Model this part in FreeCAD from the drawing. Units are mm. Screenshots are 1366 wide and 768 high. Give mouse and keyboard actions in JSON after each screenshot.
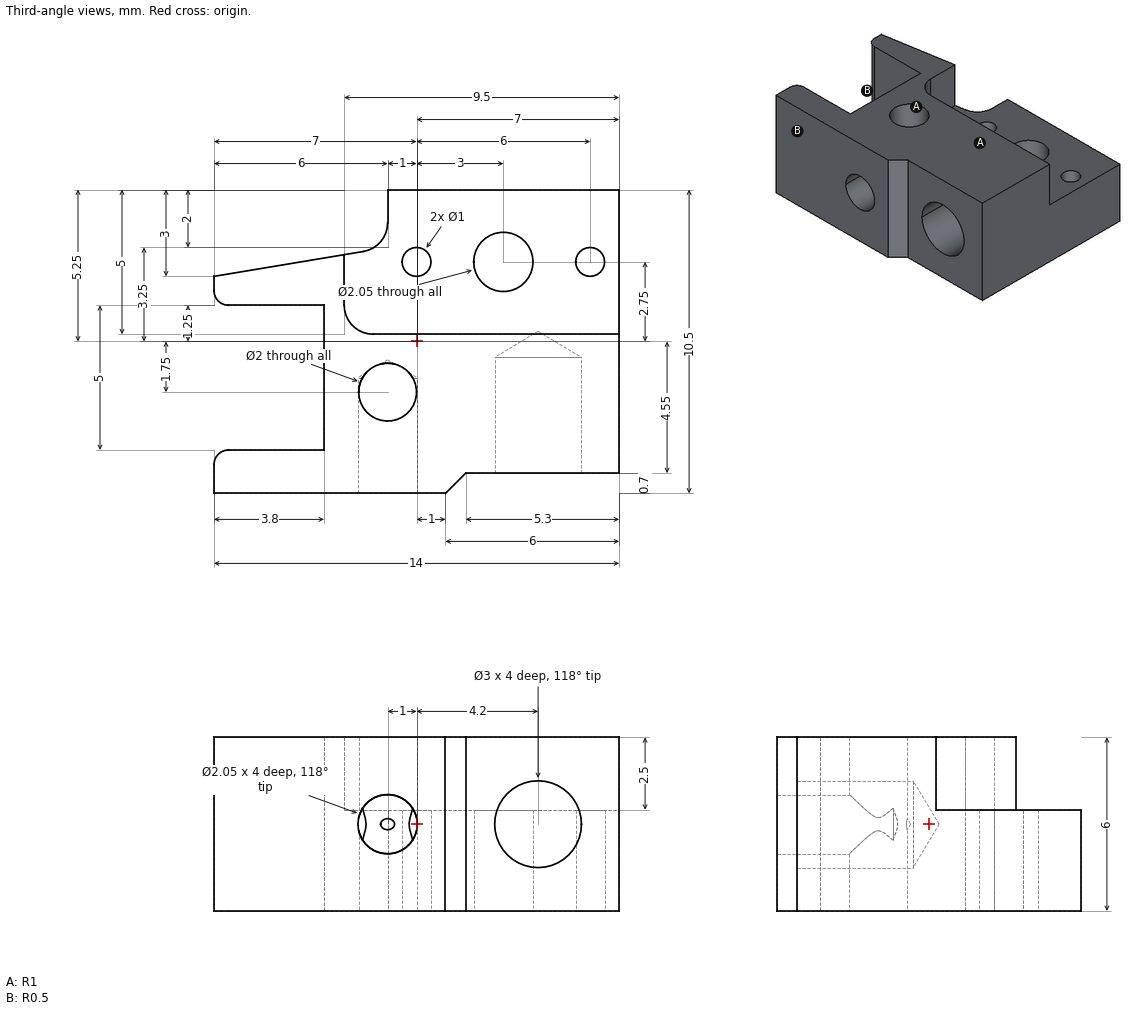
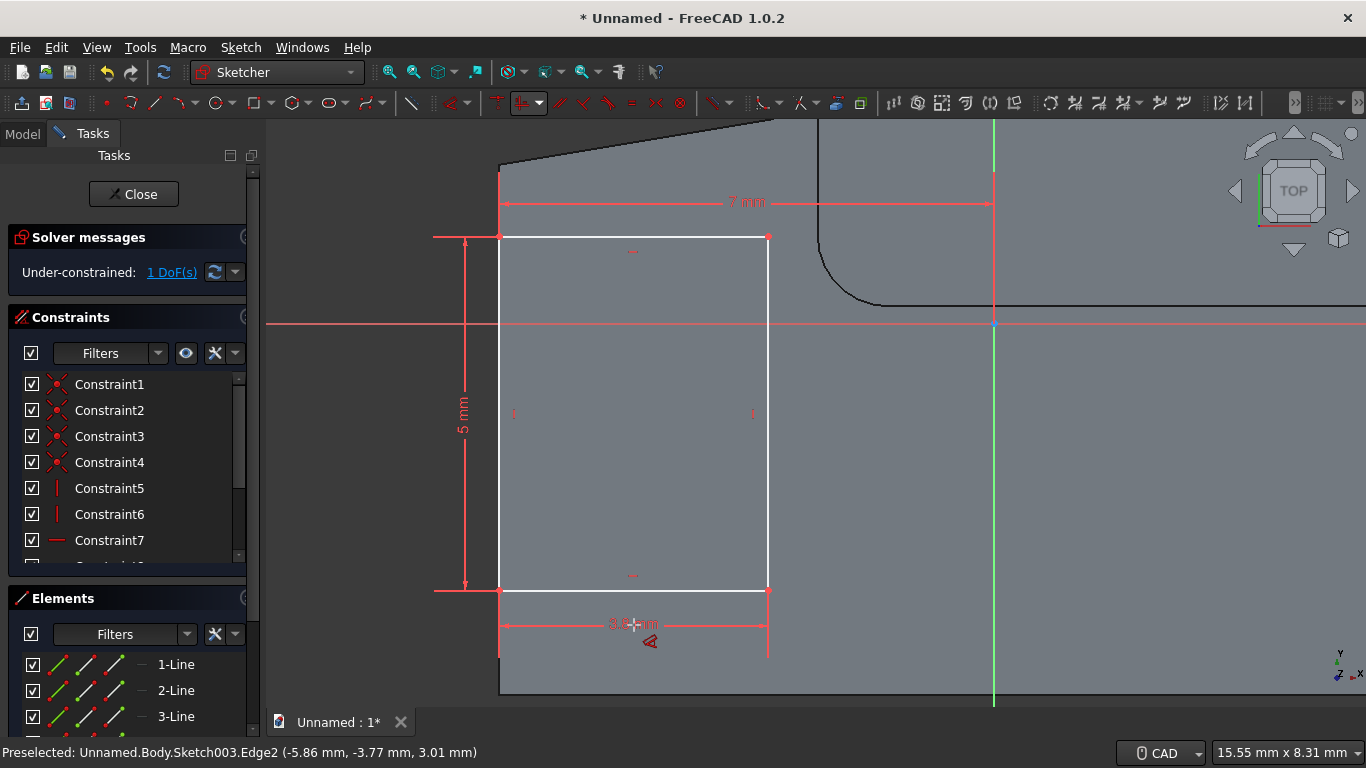
{"action": "left_click", "coordinate": [499, 237]}
{"action": "left_click", "coordinate": [1028, 280]}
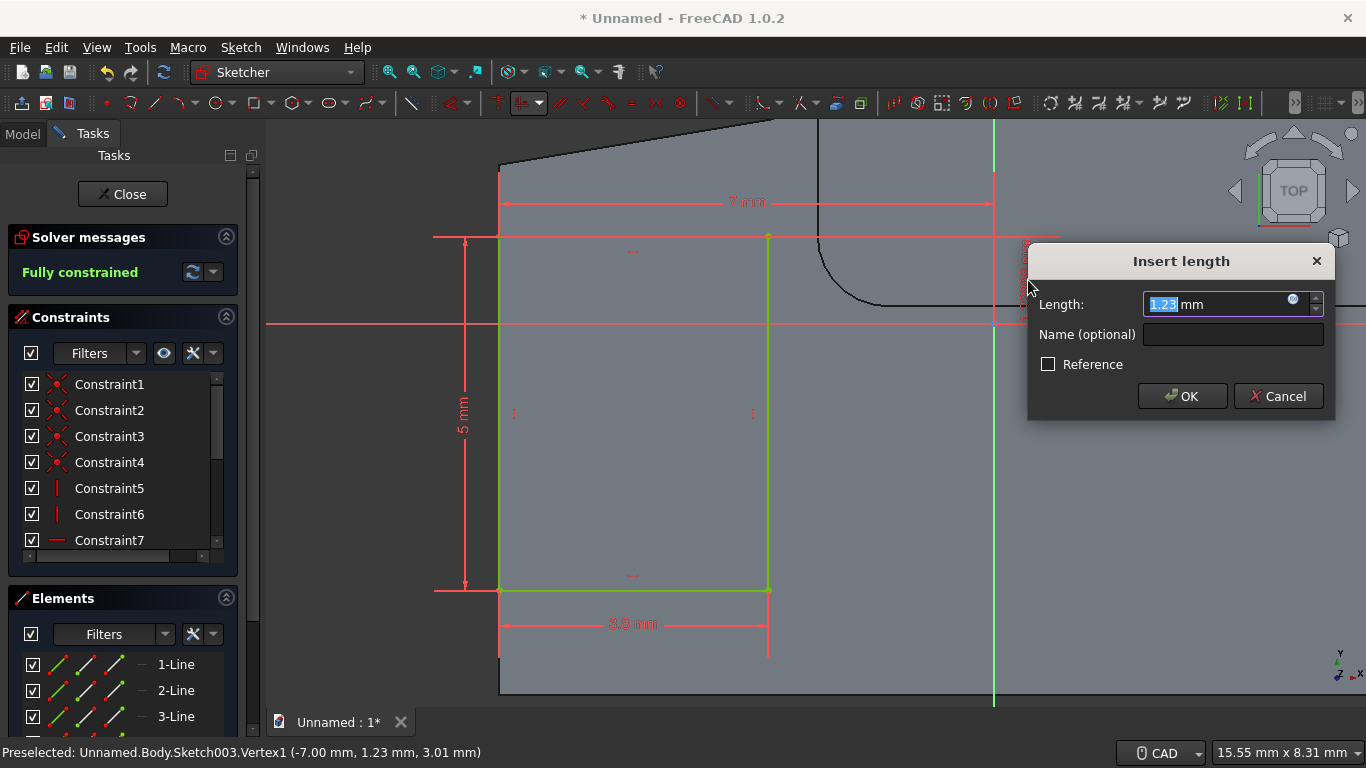
{"action": "type", "text": "1.25"}
{"action": "key", "text": "Return"}
{"action": "key", "text": "Escape"}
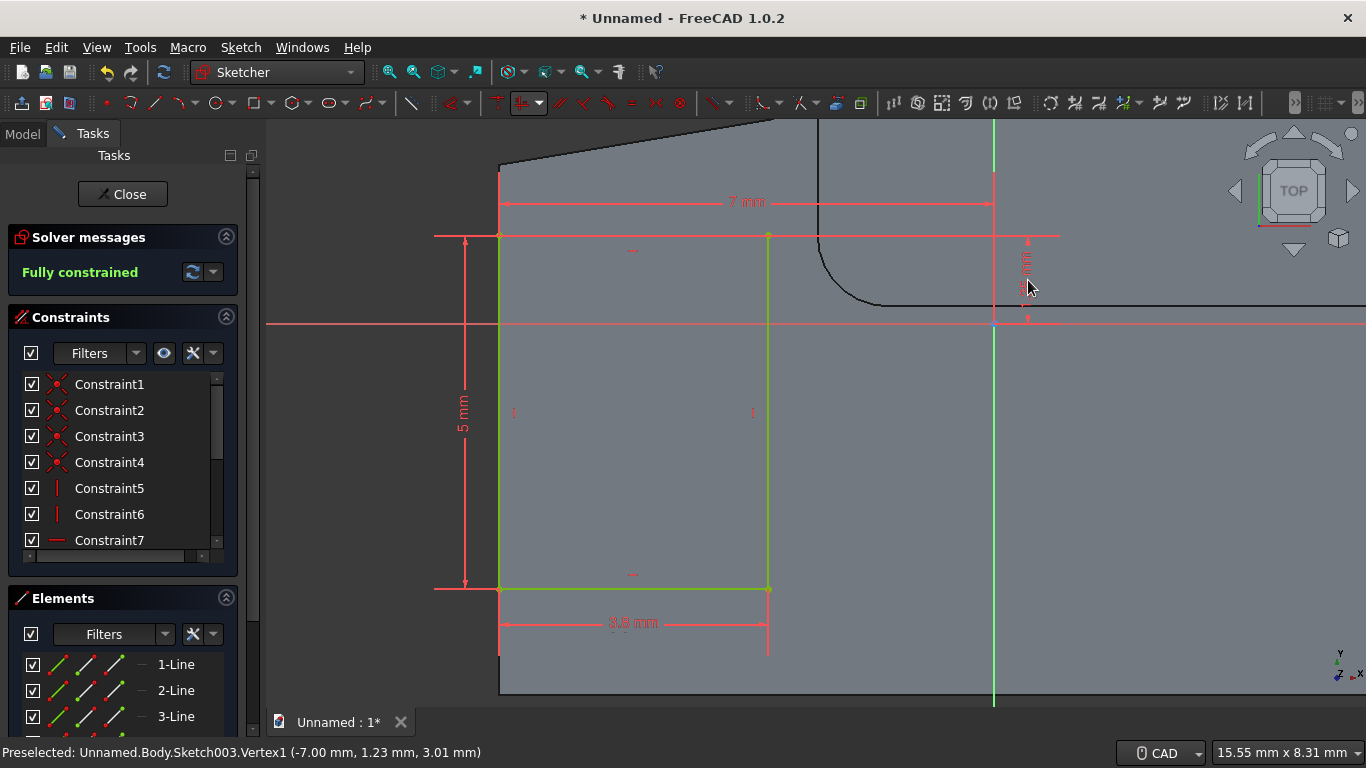
{"action": "left_click", "coordinate": [123, 194]}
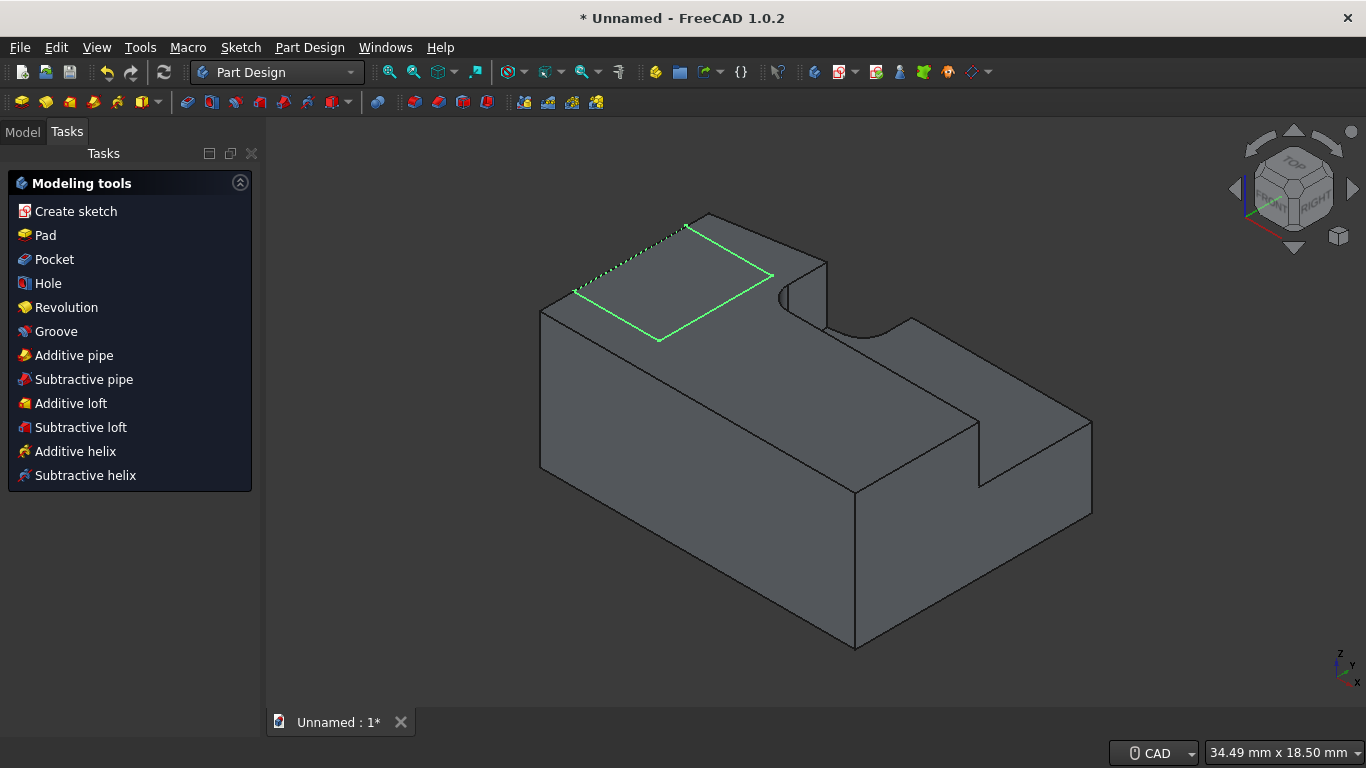
{"action": "left_click", "coordinate": [188, 102]}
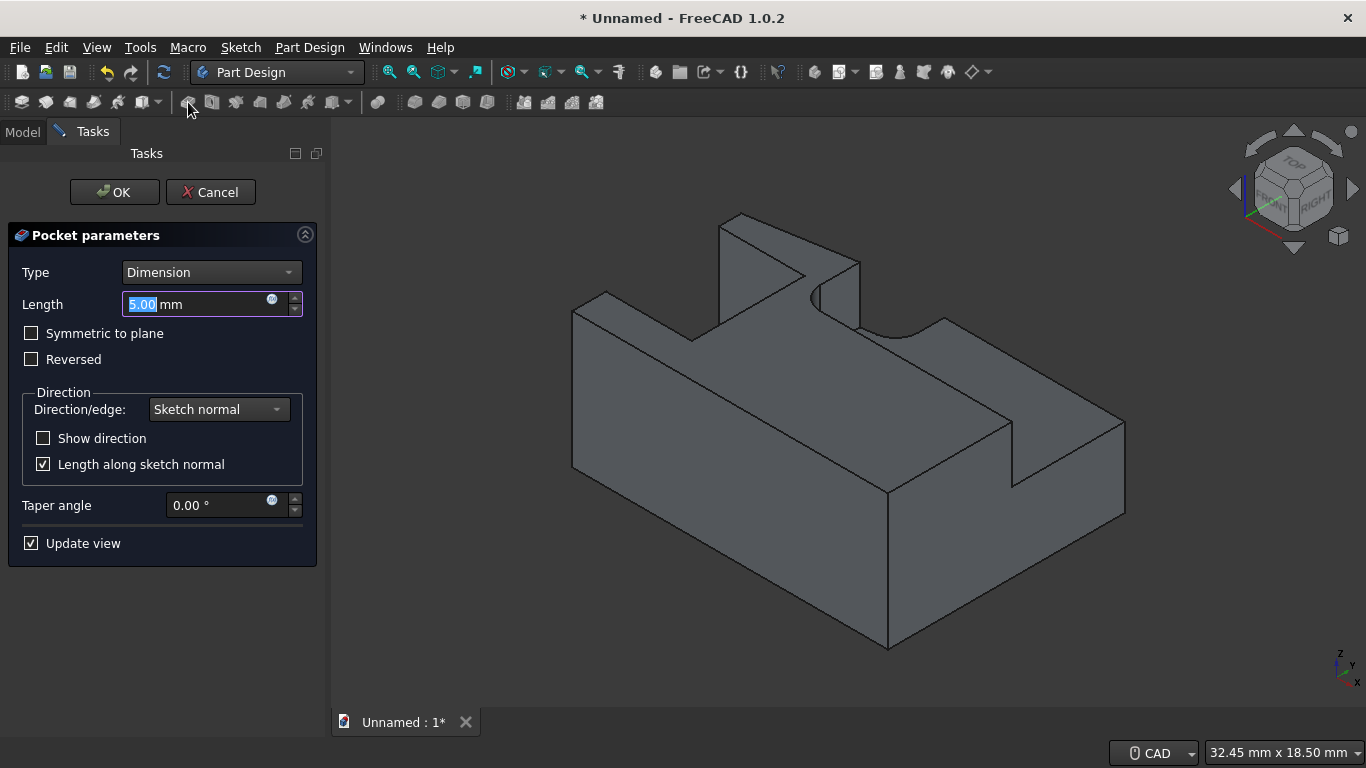
{"action": "left_click", "coordinate": [212, 272]}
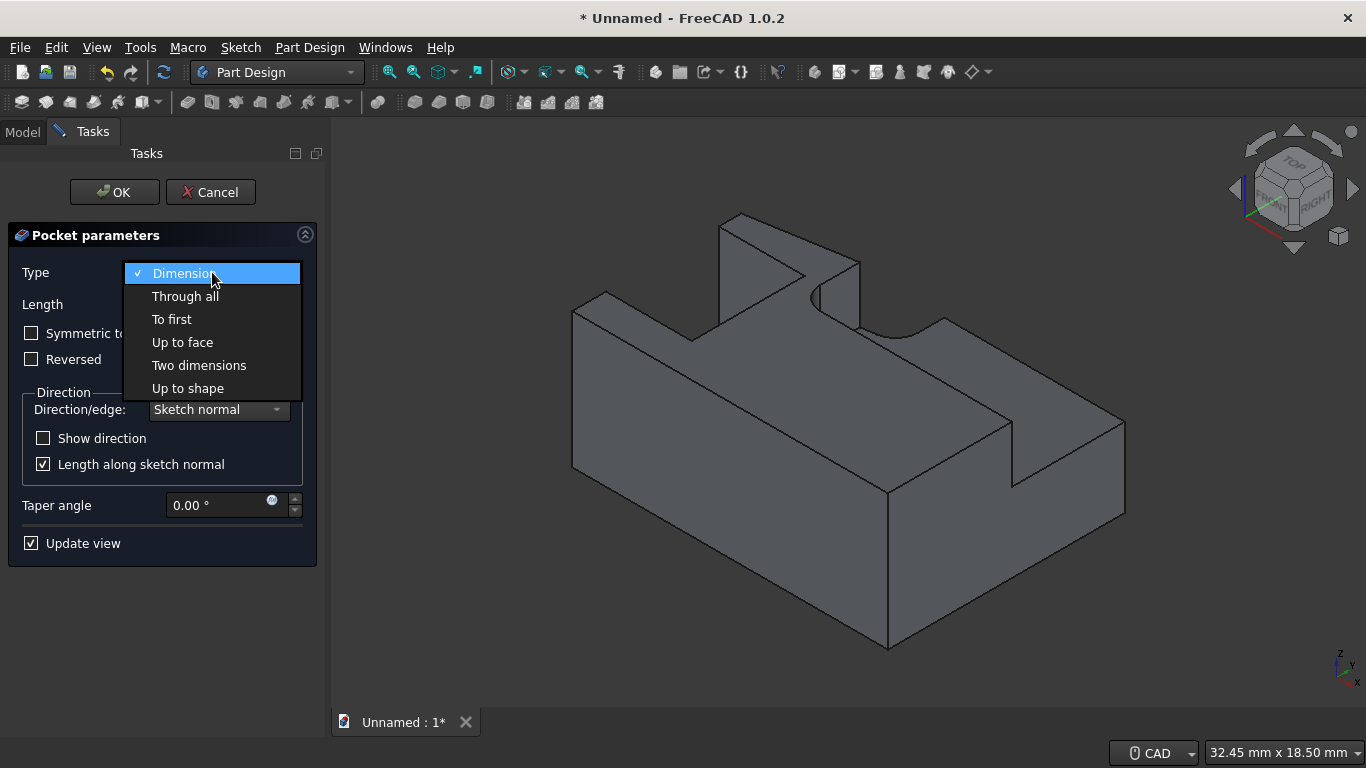
{"action": "left_click", "coordinate": [212, 296]}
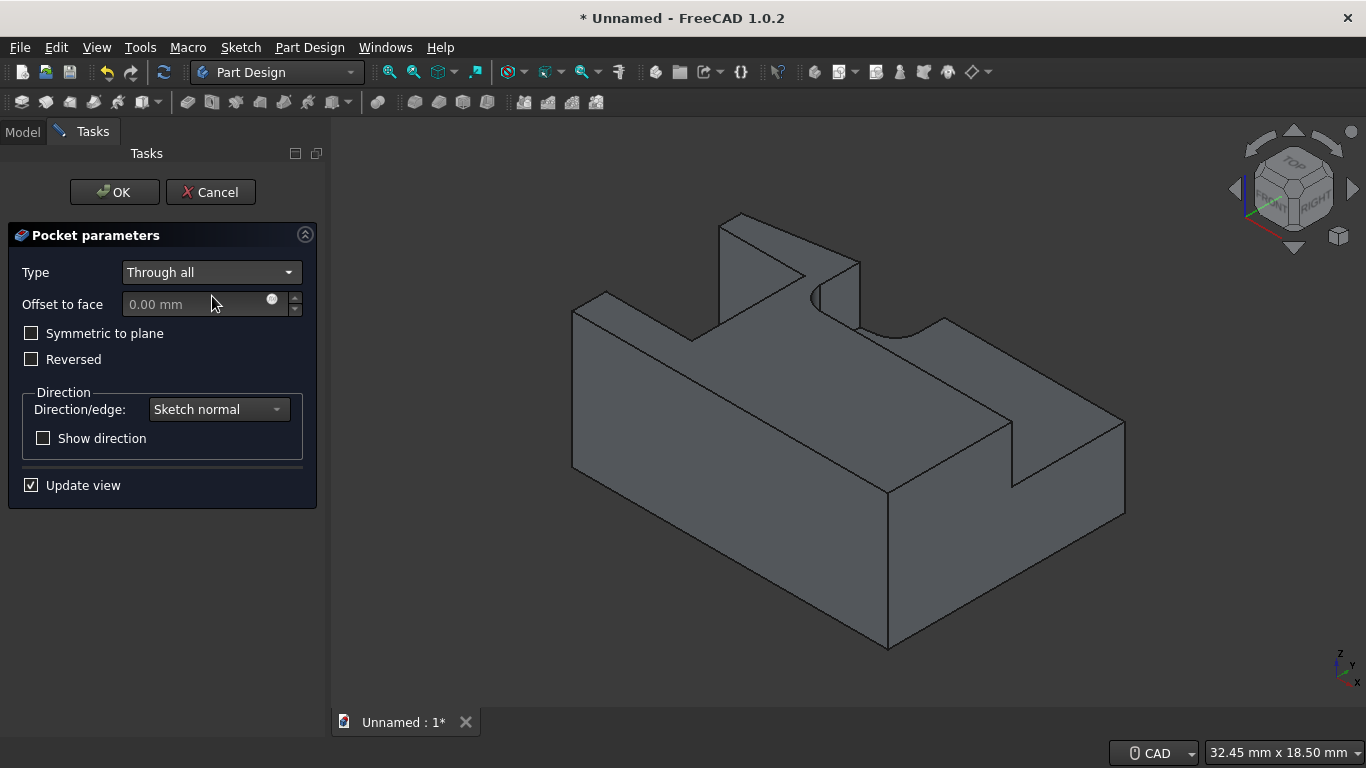
{"action": "left_click", "coordinate": [115, 192]}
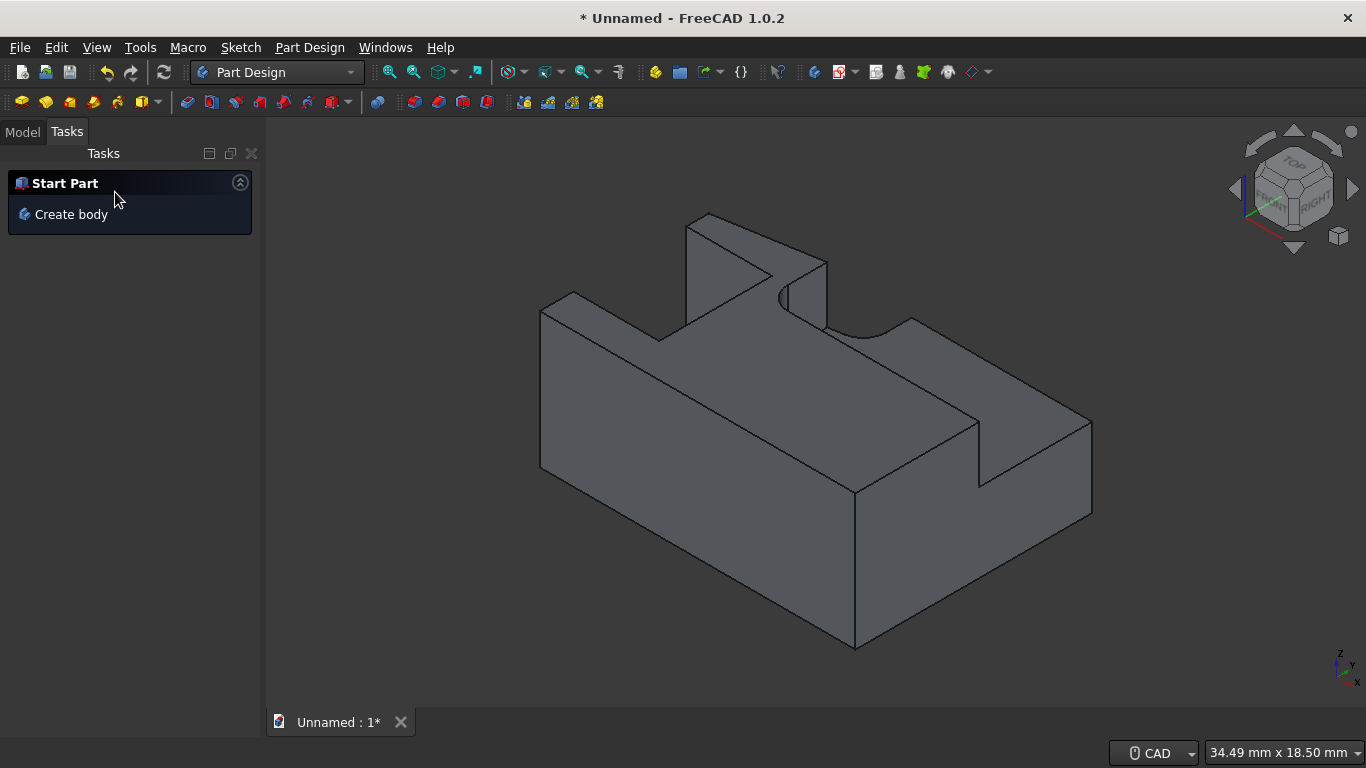
{"action": "left_click", "coordinate": [990, 427]}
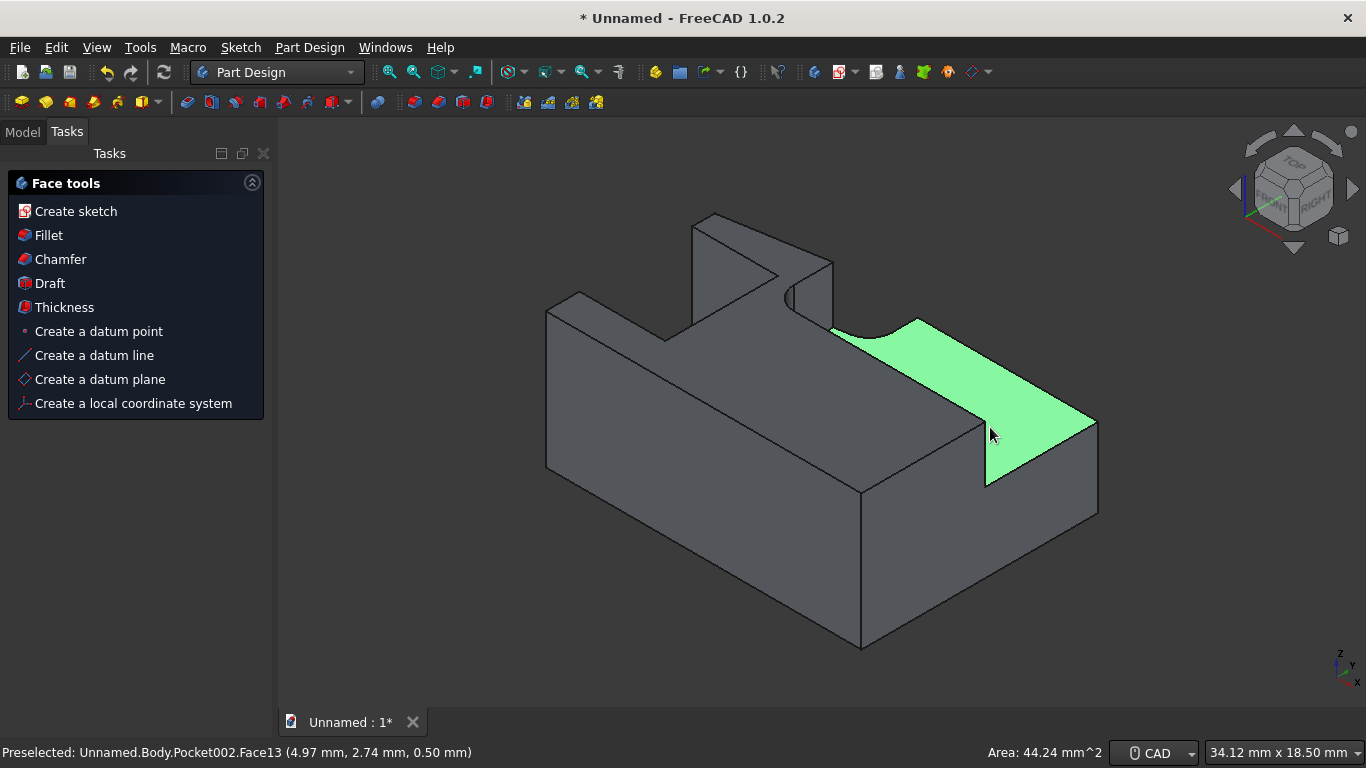
{"action": "left_click", "coordinate": [840, 72]}